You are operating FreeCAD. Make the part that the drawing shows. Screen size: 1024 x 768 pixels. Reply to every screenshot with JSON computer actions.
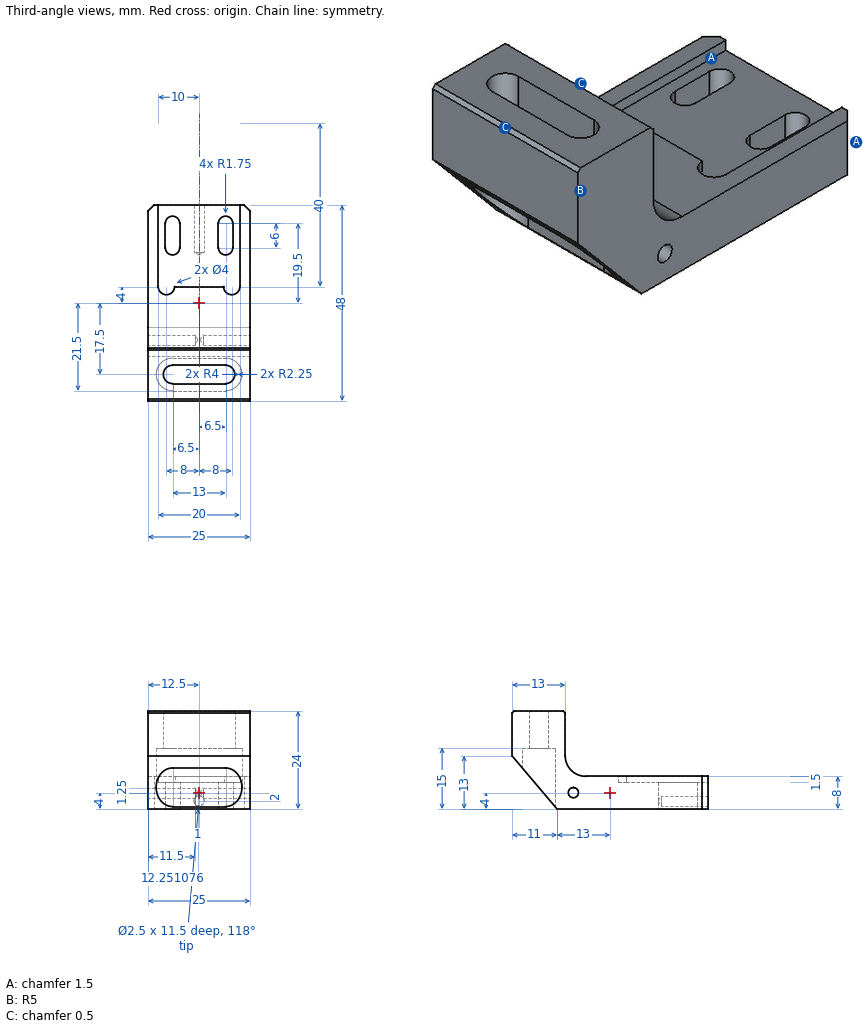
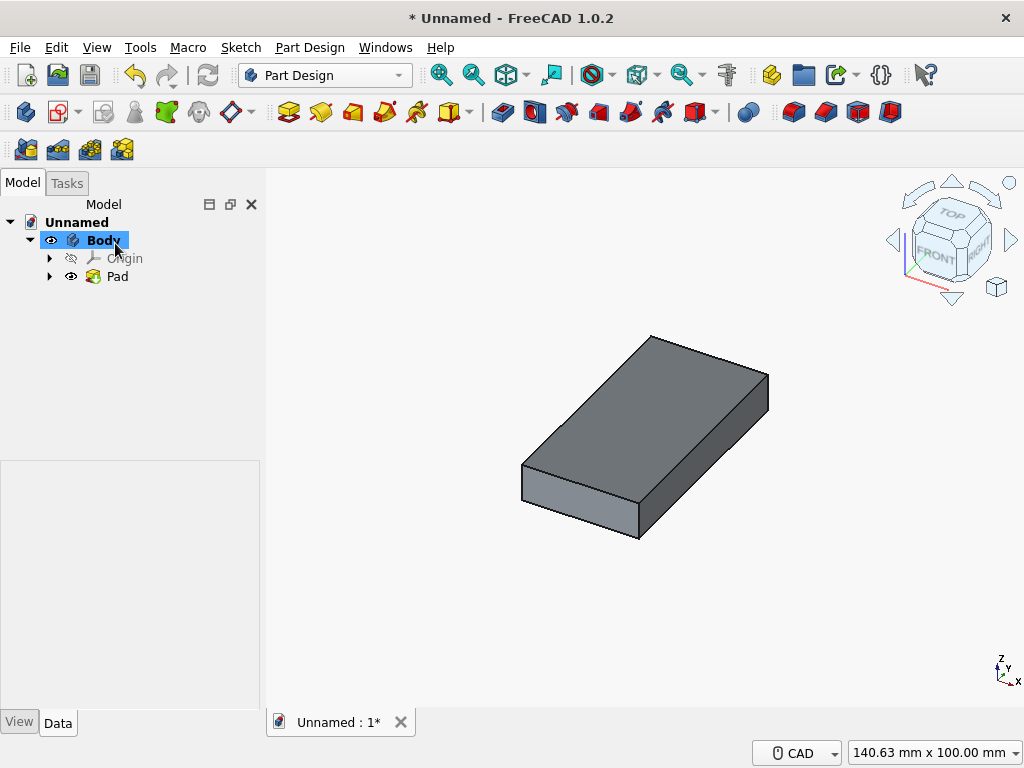
{"action": "left_click", "coordinate": [442, 76]}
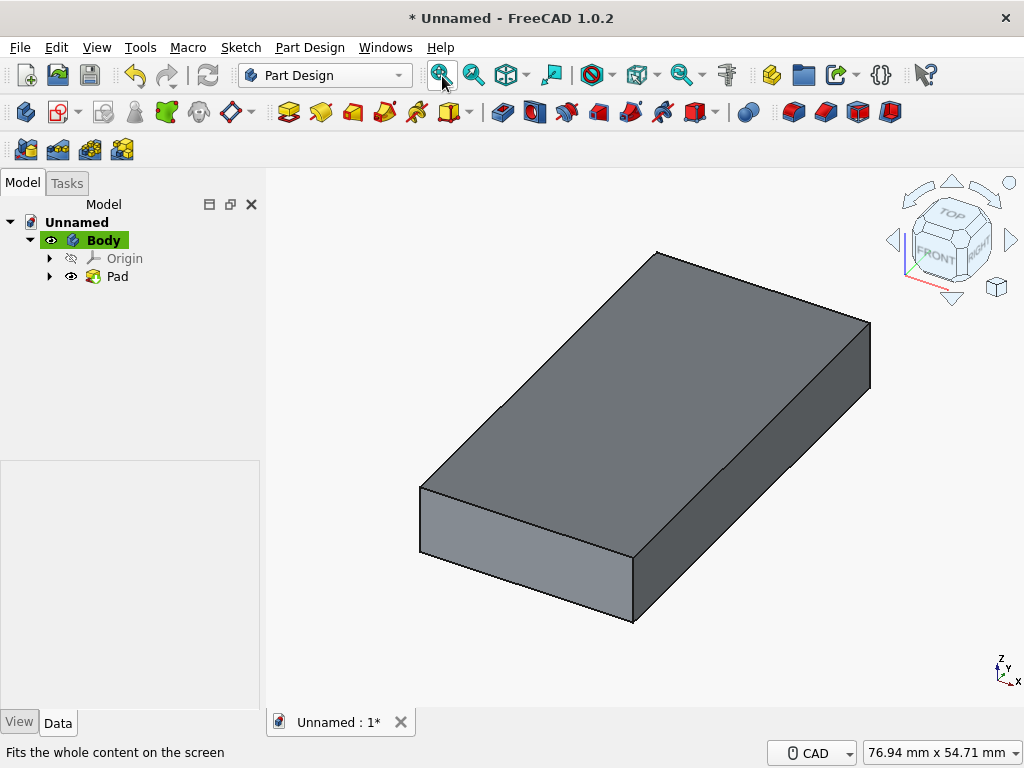
{"action": "left_click", "coordinate": [588, 574]}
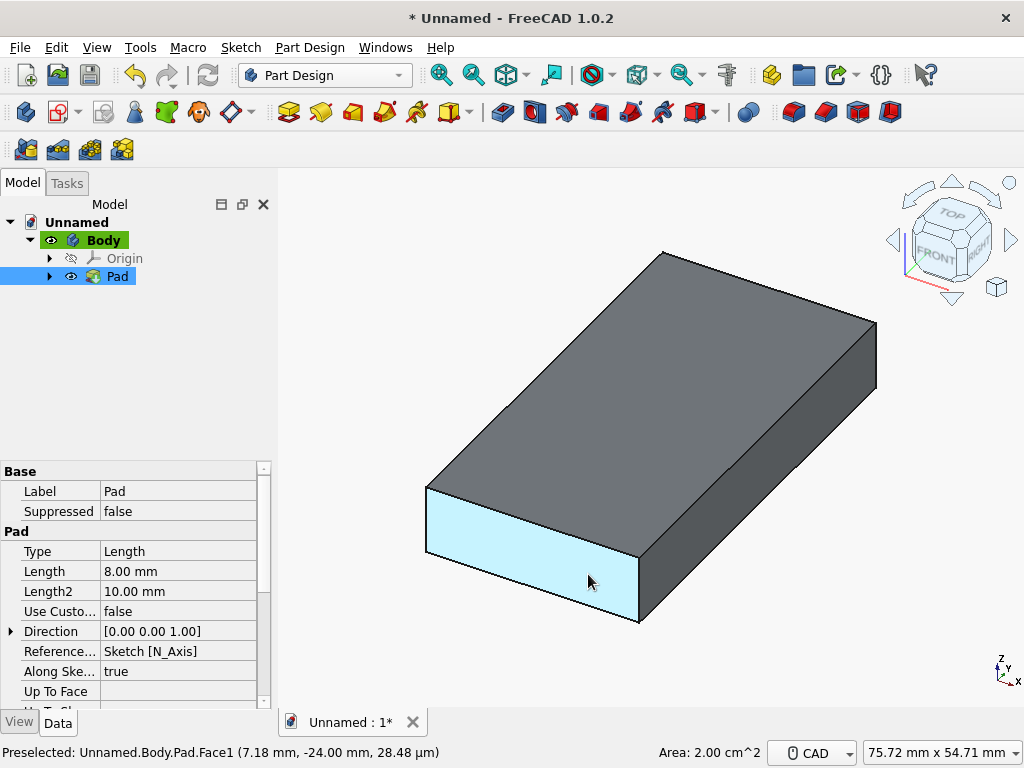
{"action": "left_click", "coordinate": [58, 112]}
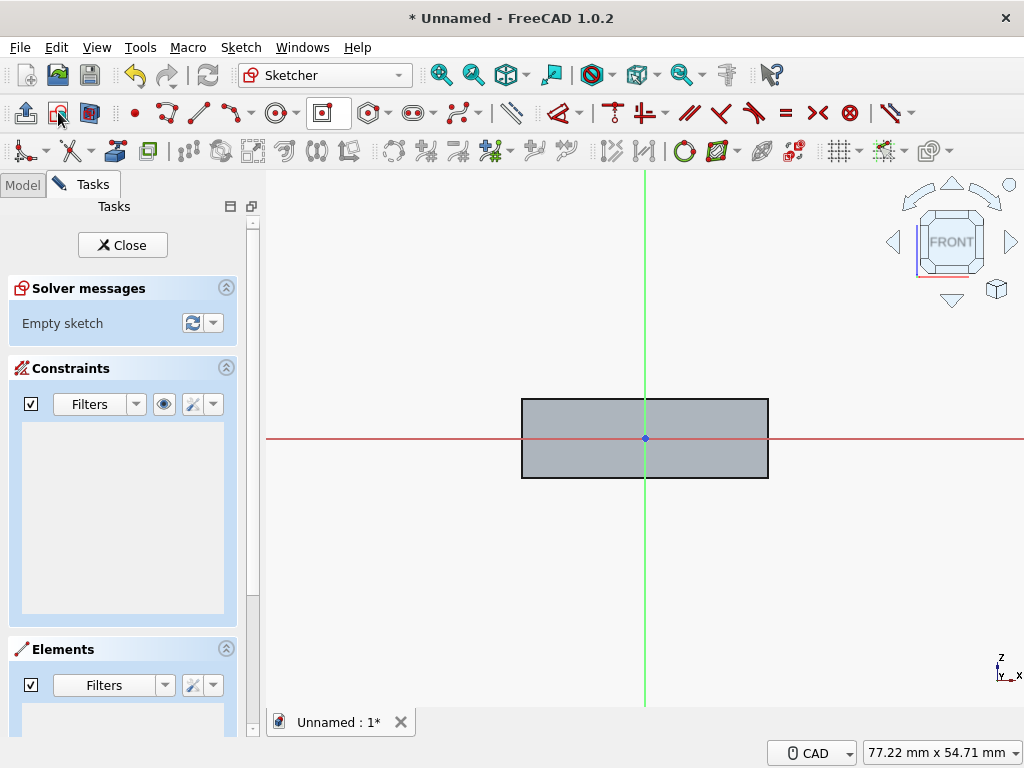
{"action": "scroll", "coordinate": [784, 200], "scroll_direction": "up", "scroll_amount": 2}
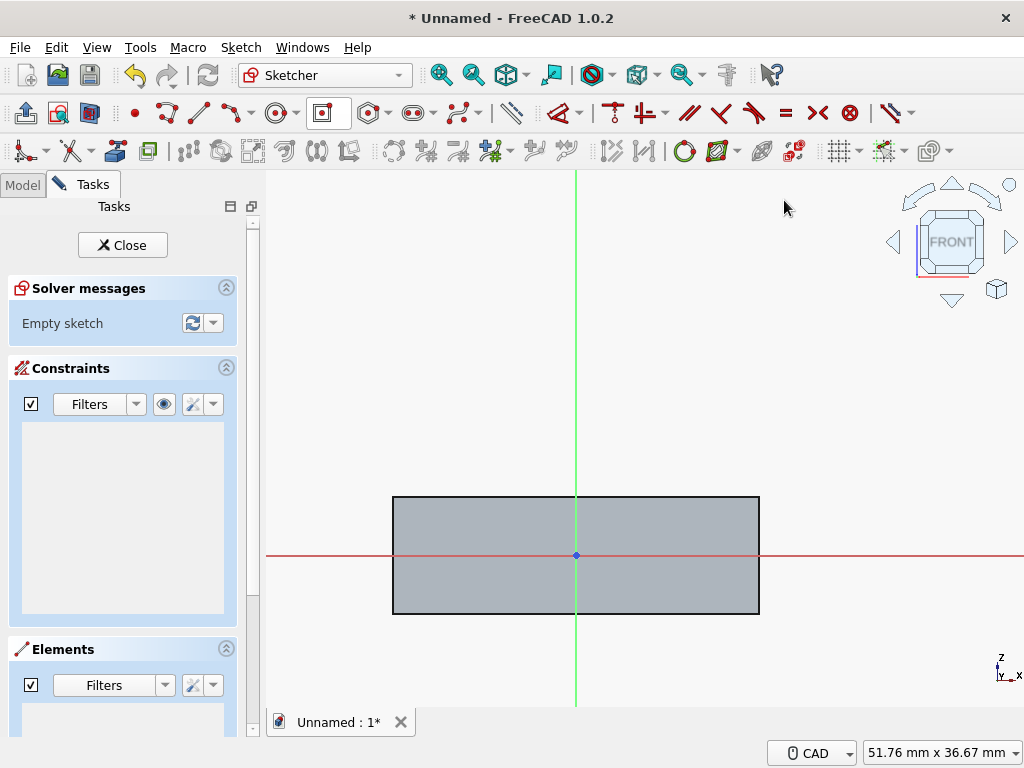
{"action": "key", "text": "g r"}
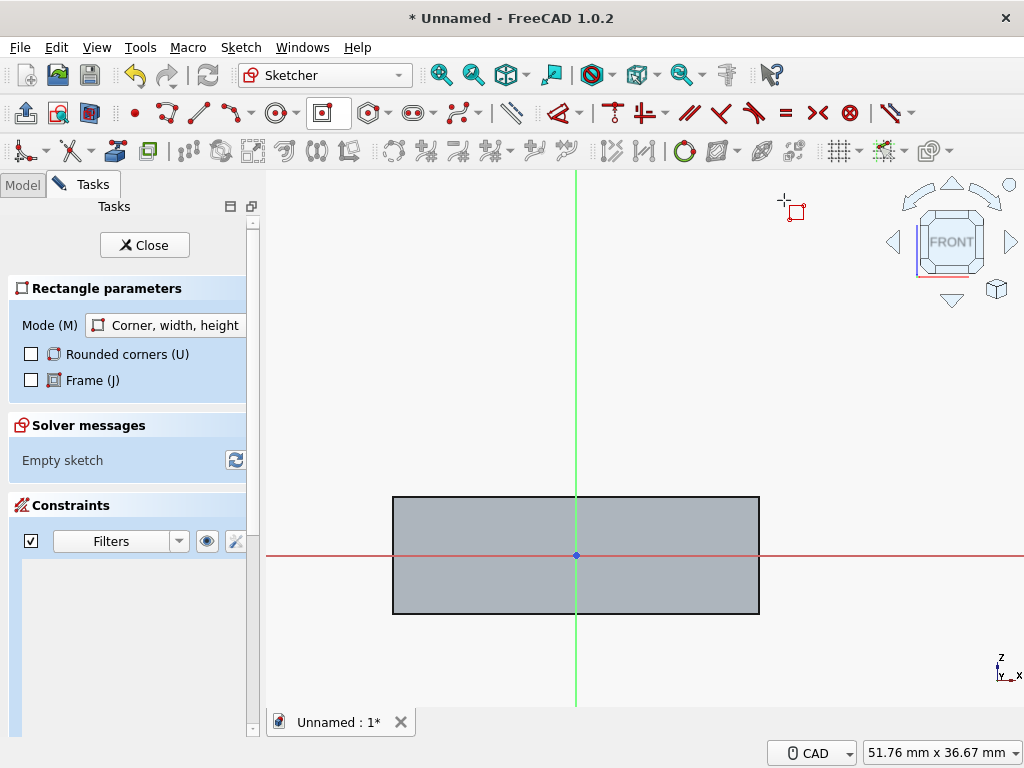
{"action": "left_click", "coordinate": [393, 263]}
{"action": "mouse_move", "coordinate": [759, 614]}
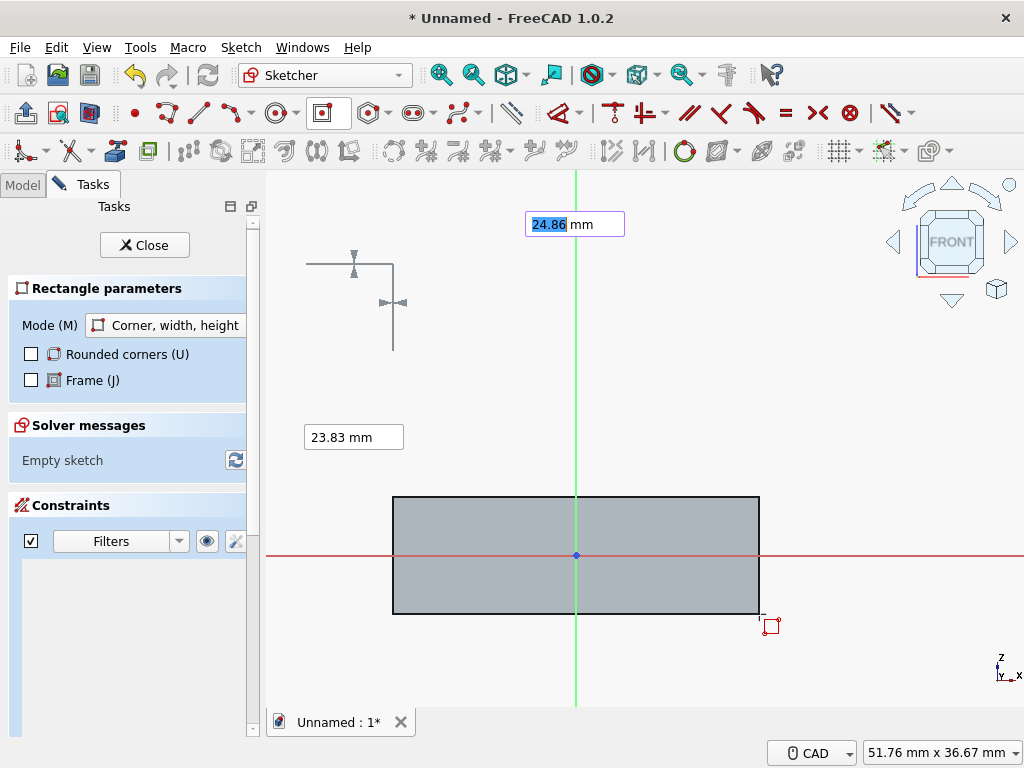
{"action": "type", "text": "25"}
{"action": "key", "text": "Tab"}
{"action": "type", "text": "24"}
{"action": "key", "text": "Return"}
{"action": "key", "text": "Escape"}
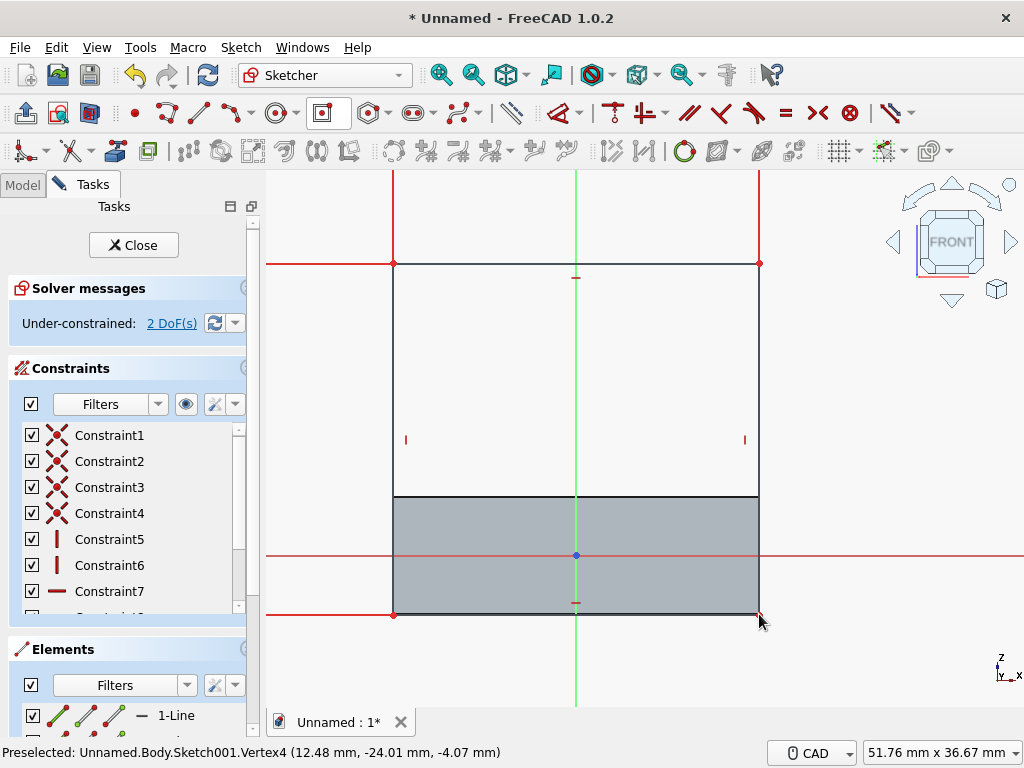
{"action": "left_click", "coordinate": [393, 615]}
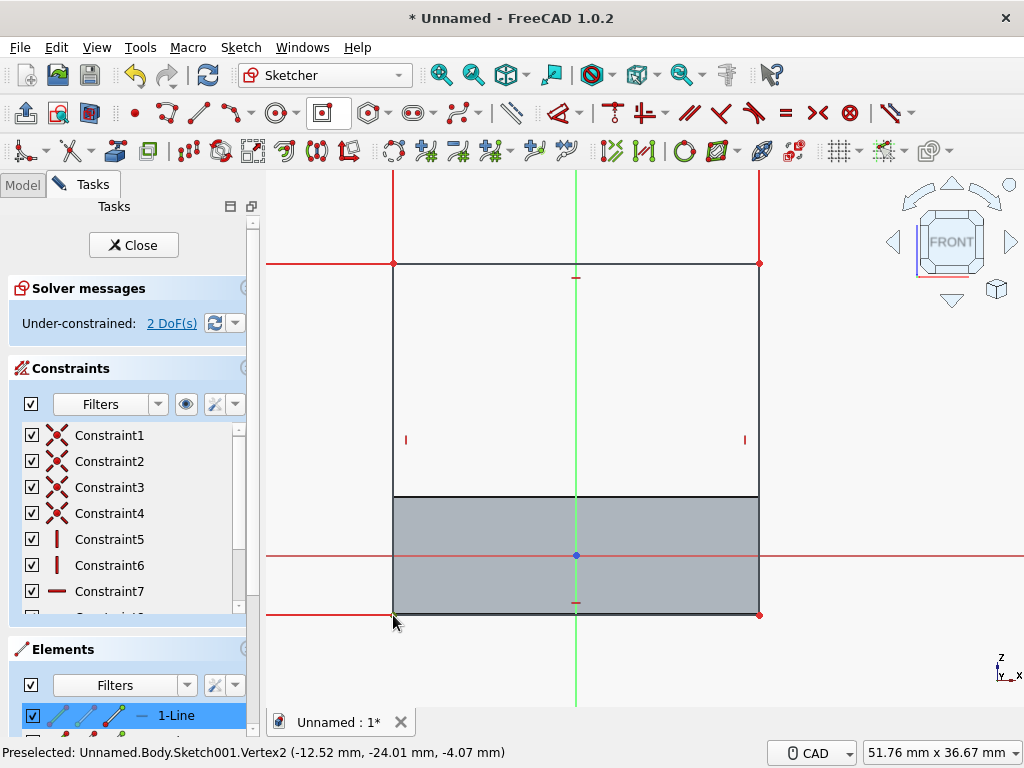
{"action": "left_click", "coordinate": [582, 114]}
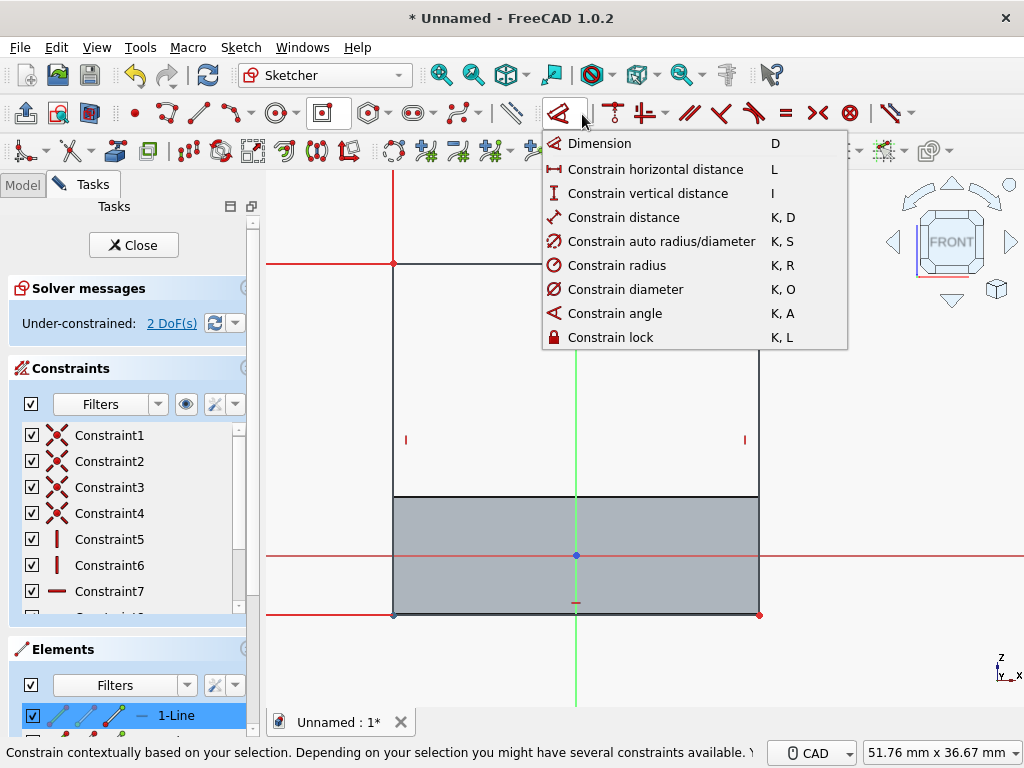
{"action": "left_click", "coordinate": [695, 193]}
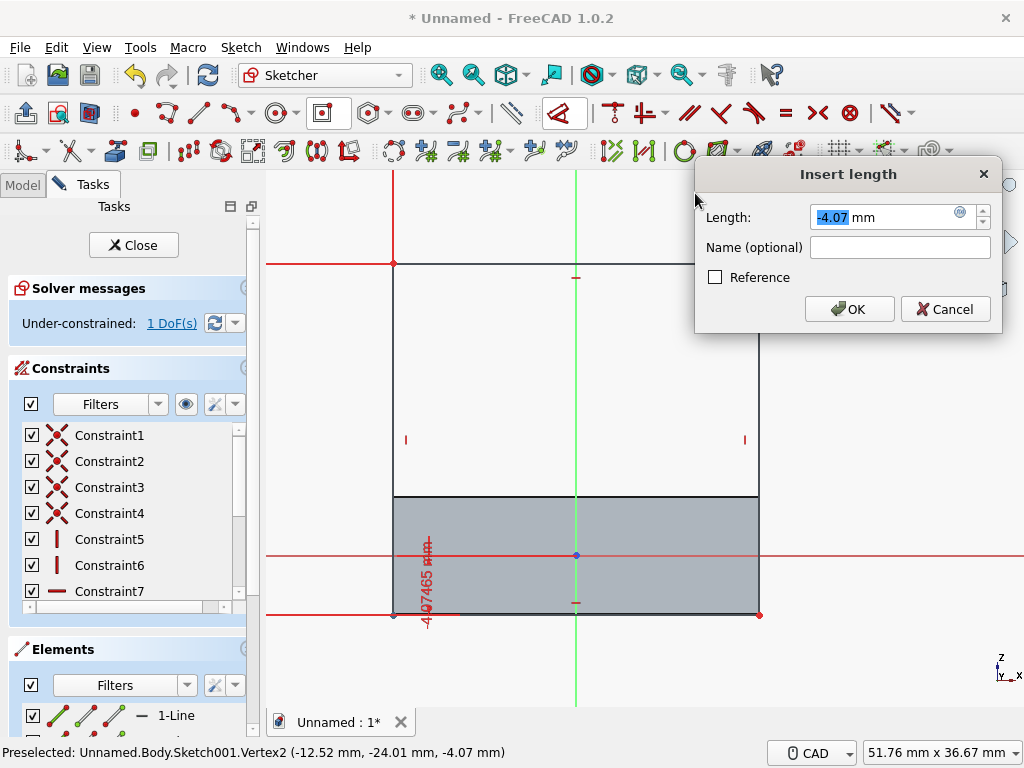
{"action": "type", "text": "-4"}
{"action": "key", "text": "Return"}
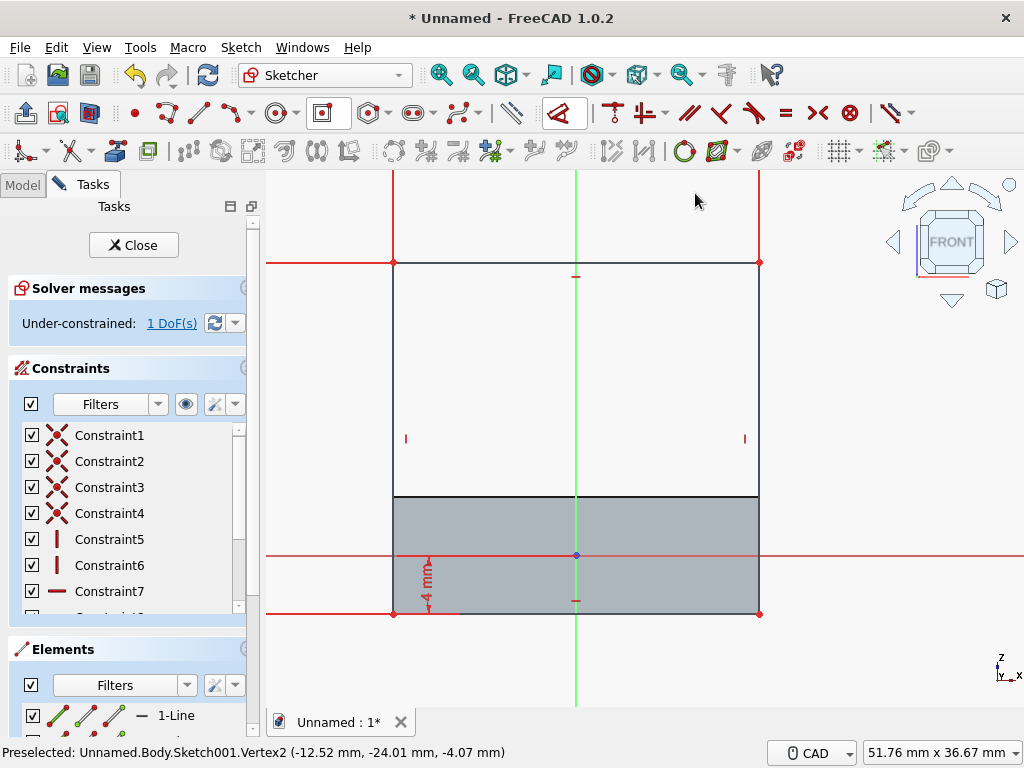
{"action": "left_click", "coordinate": [393, 263]}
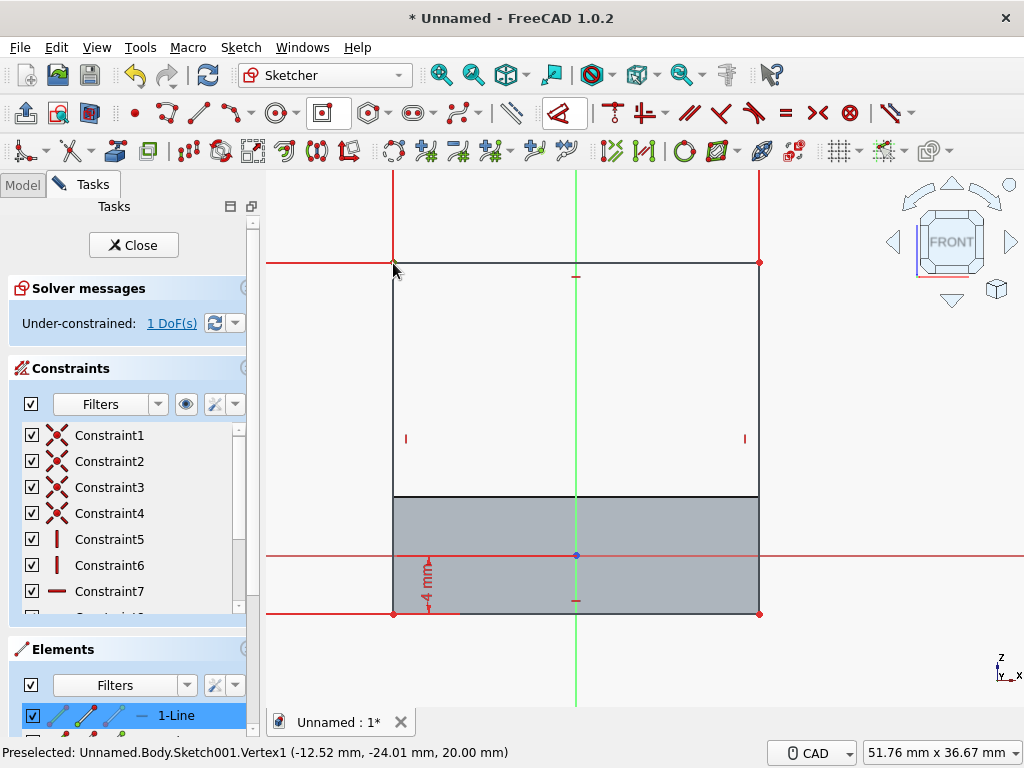
{"action": "left_click", "coordinate": [582, 114]}